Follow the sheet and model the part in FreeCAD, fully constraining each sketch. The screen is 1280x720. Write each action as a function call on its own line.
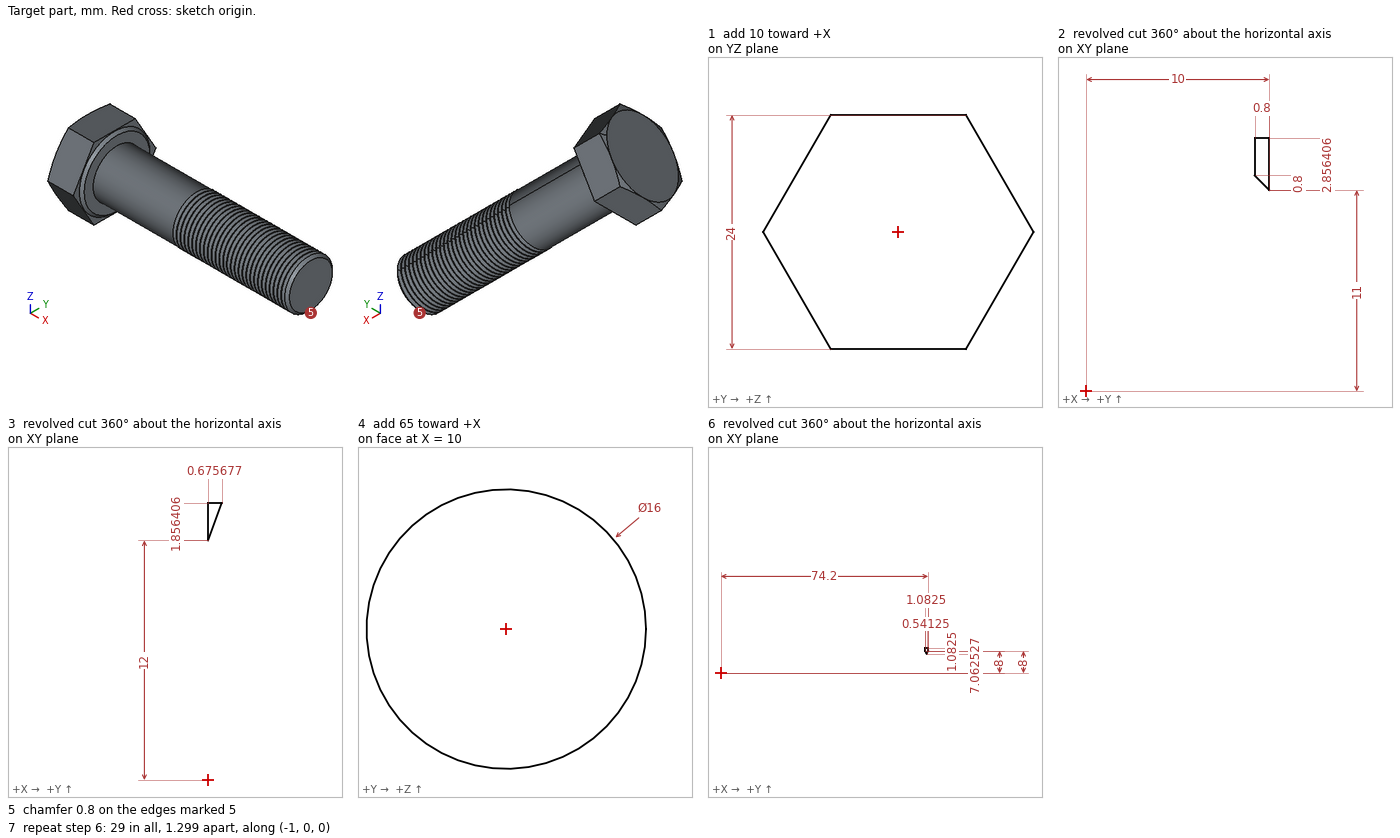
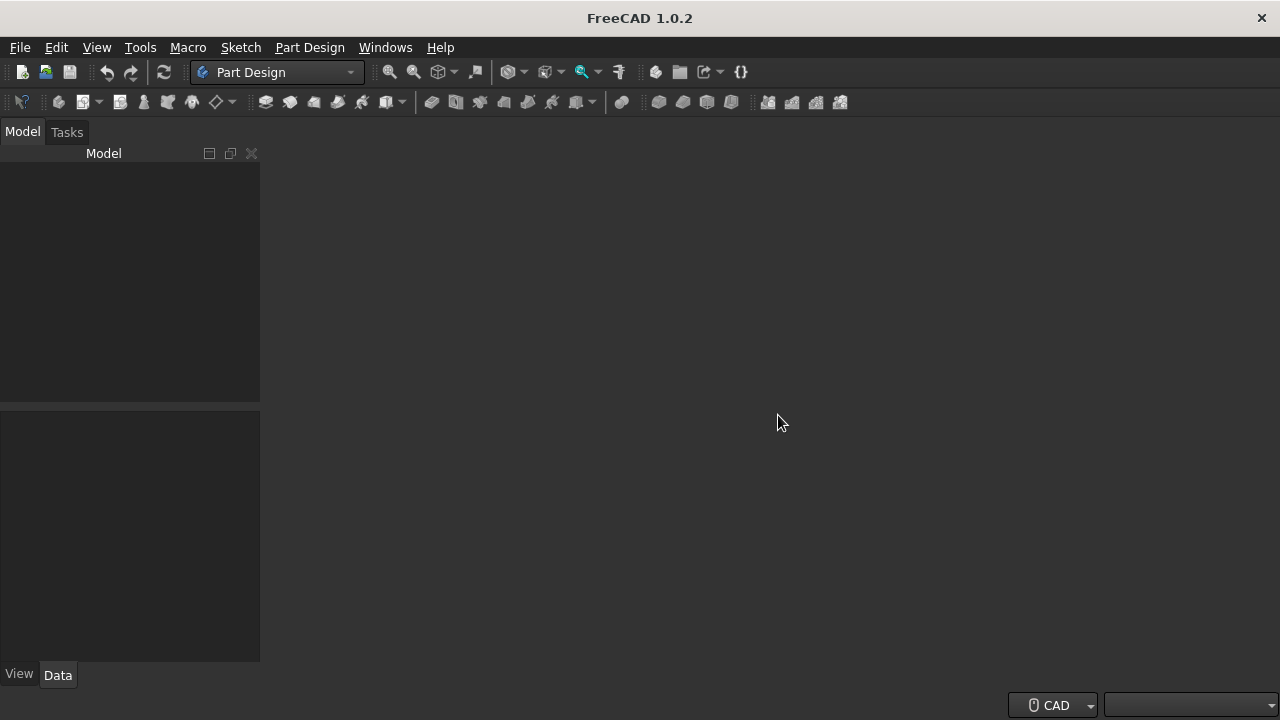
click(22, 72)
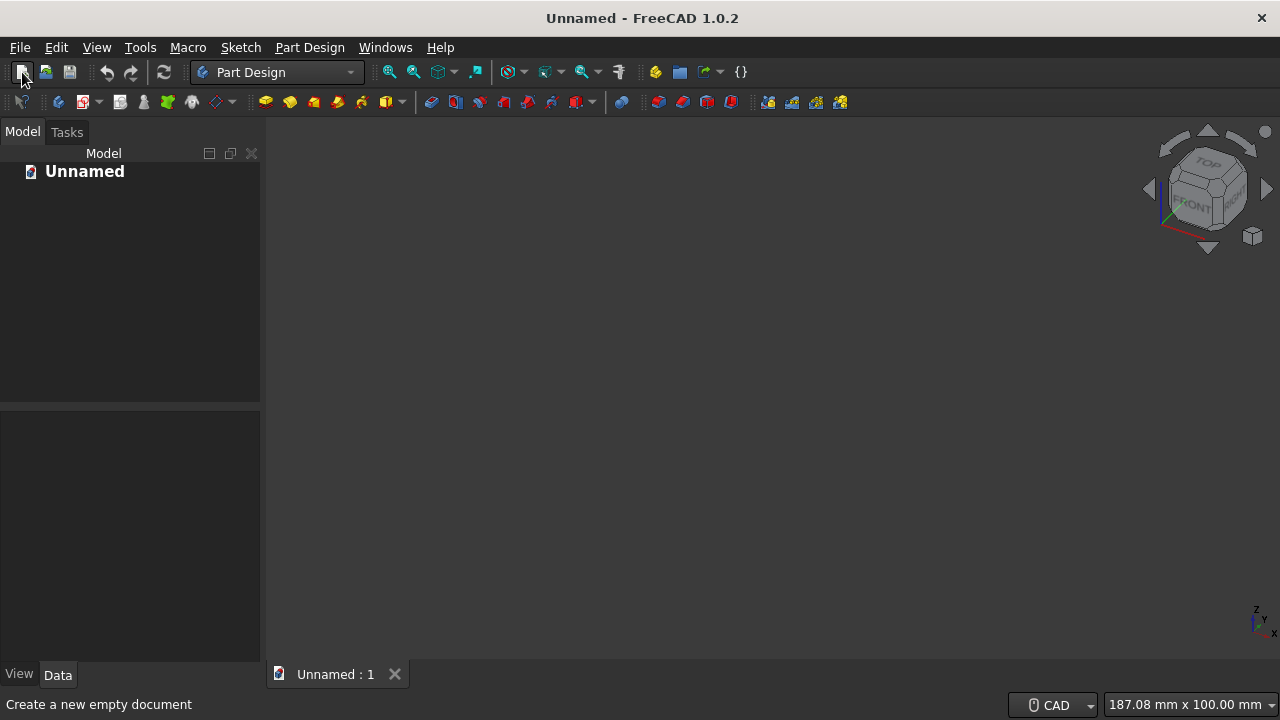
click(84, 102)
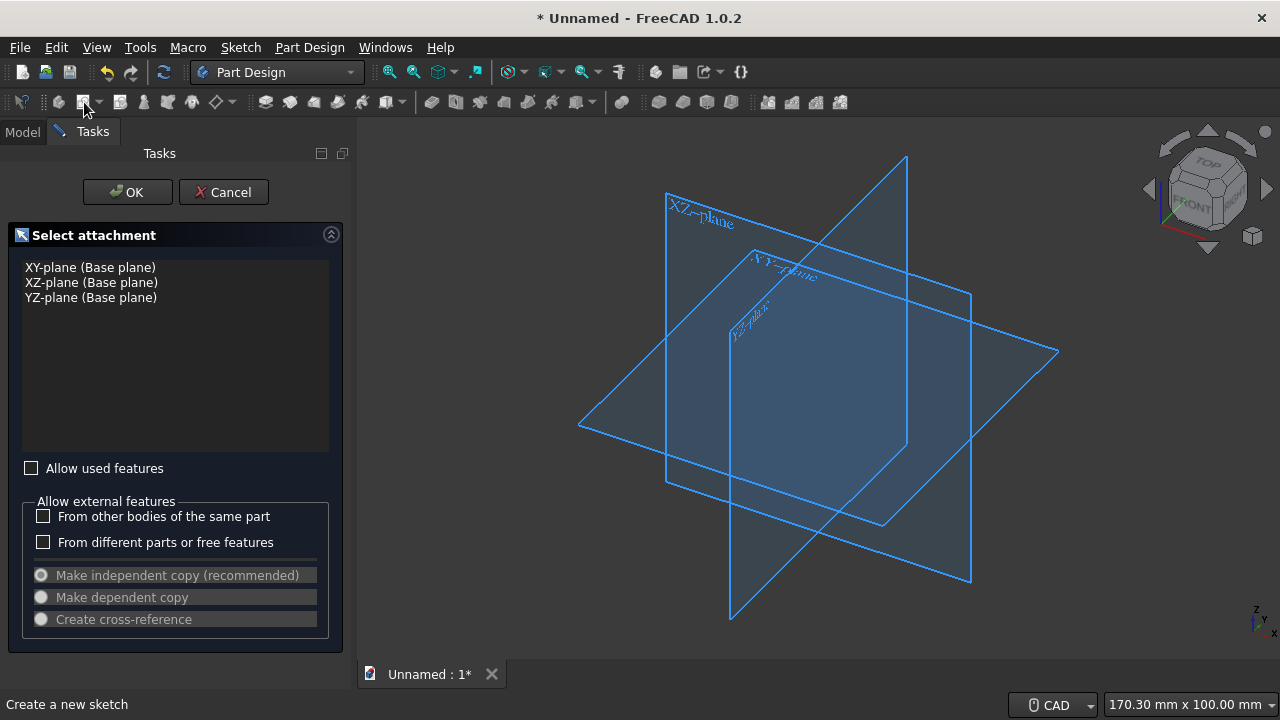
click(82, 298)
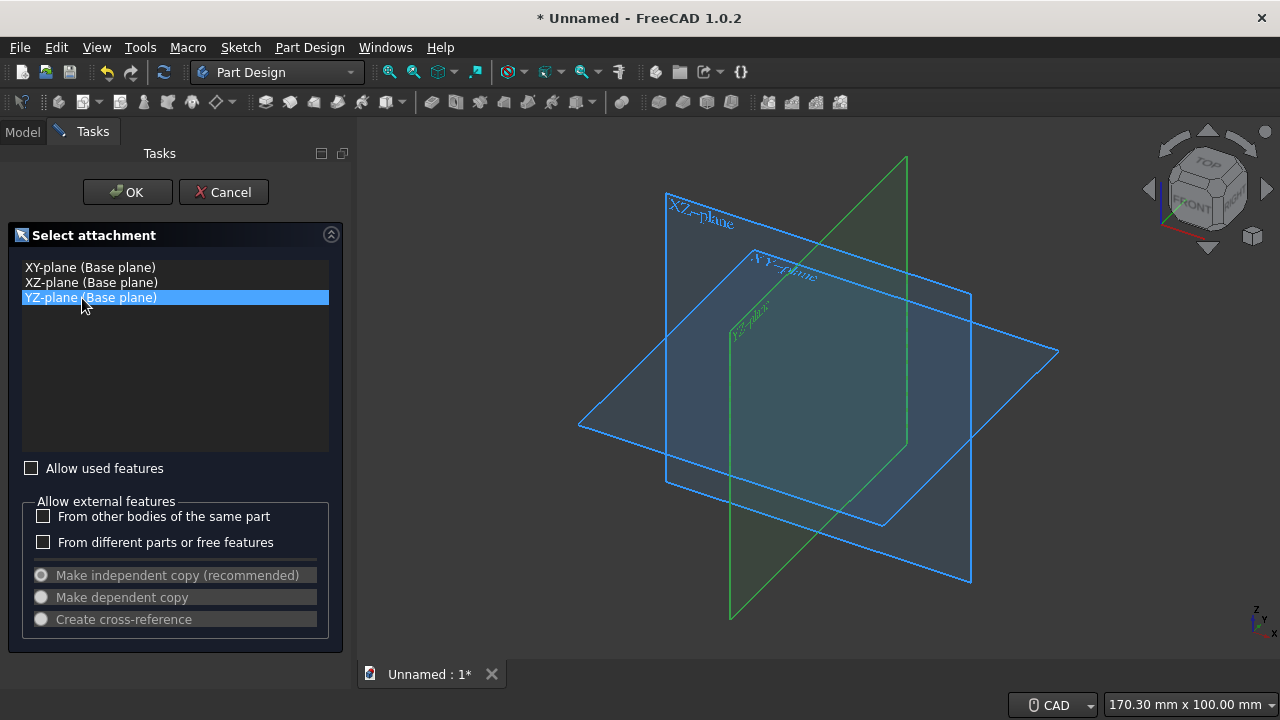
click(128, 192)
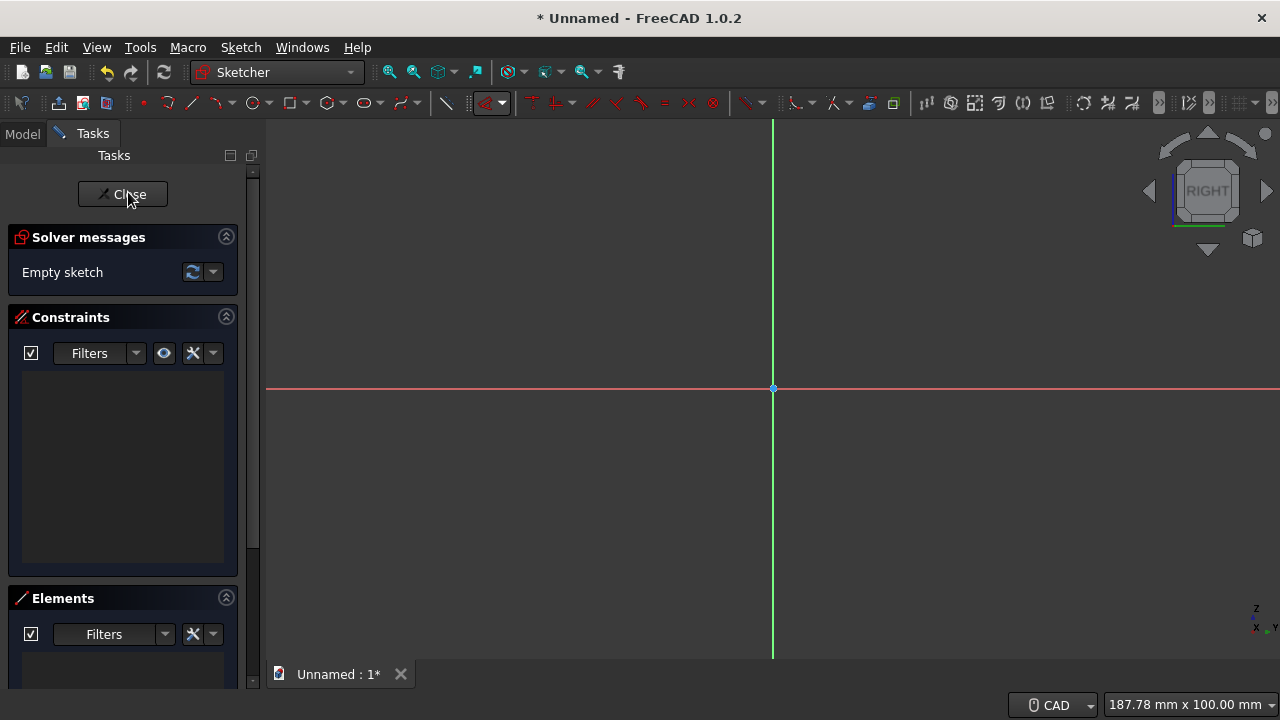
scroll(813, 389, up, 5)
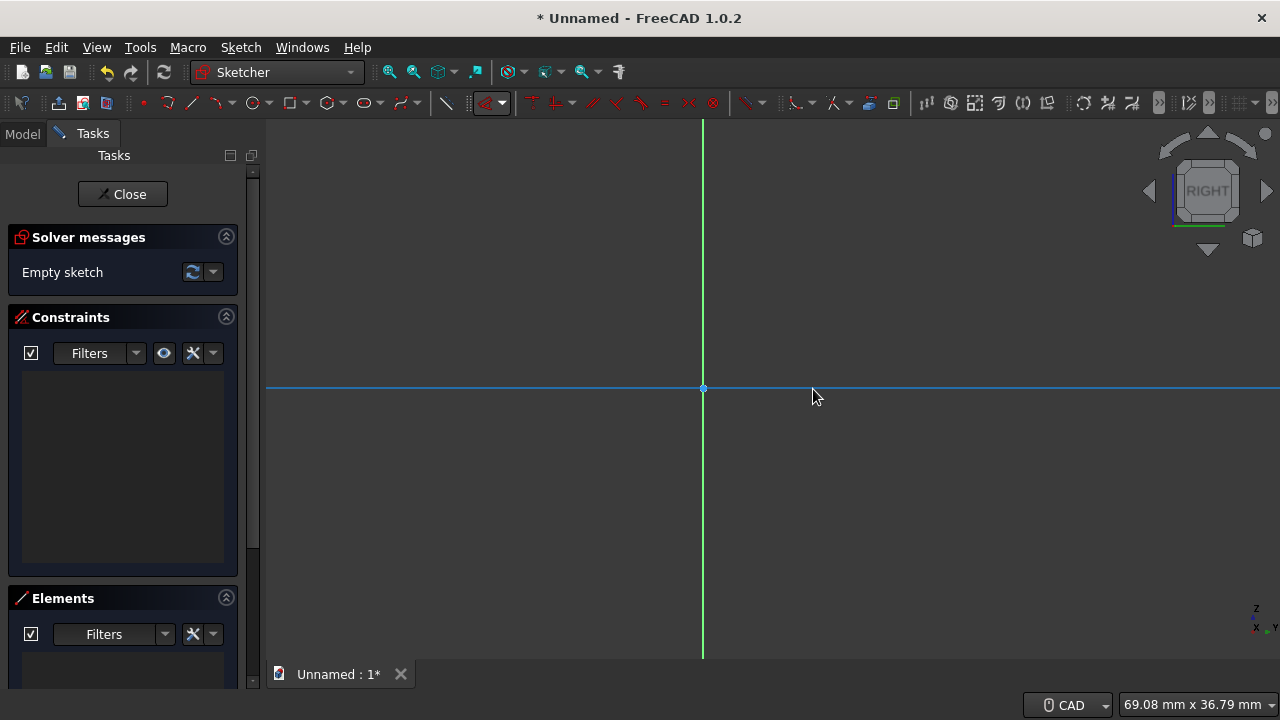
key(g)
key(p)
key(6)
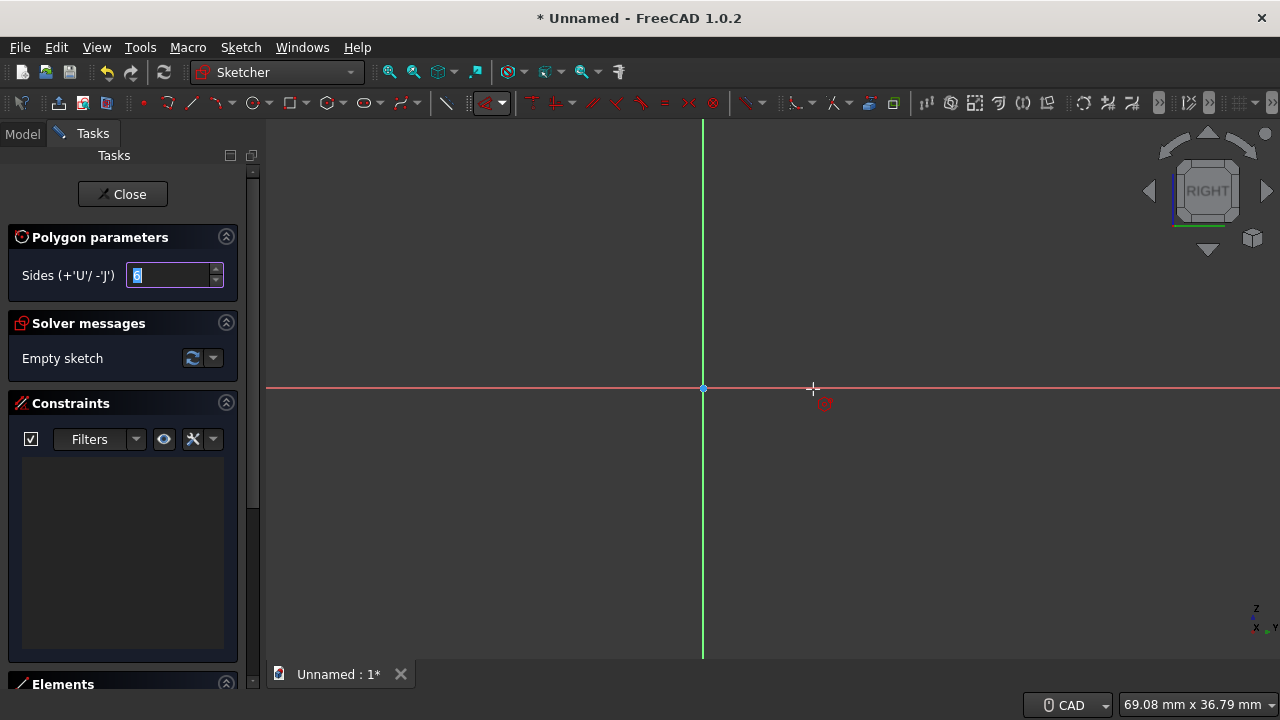
click(703, 388)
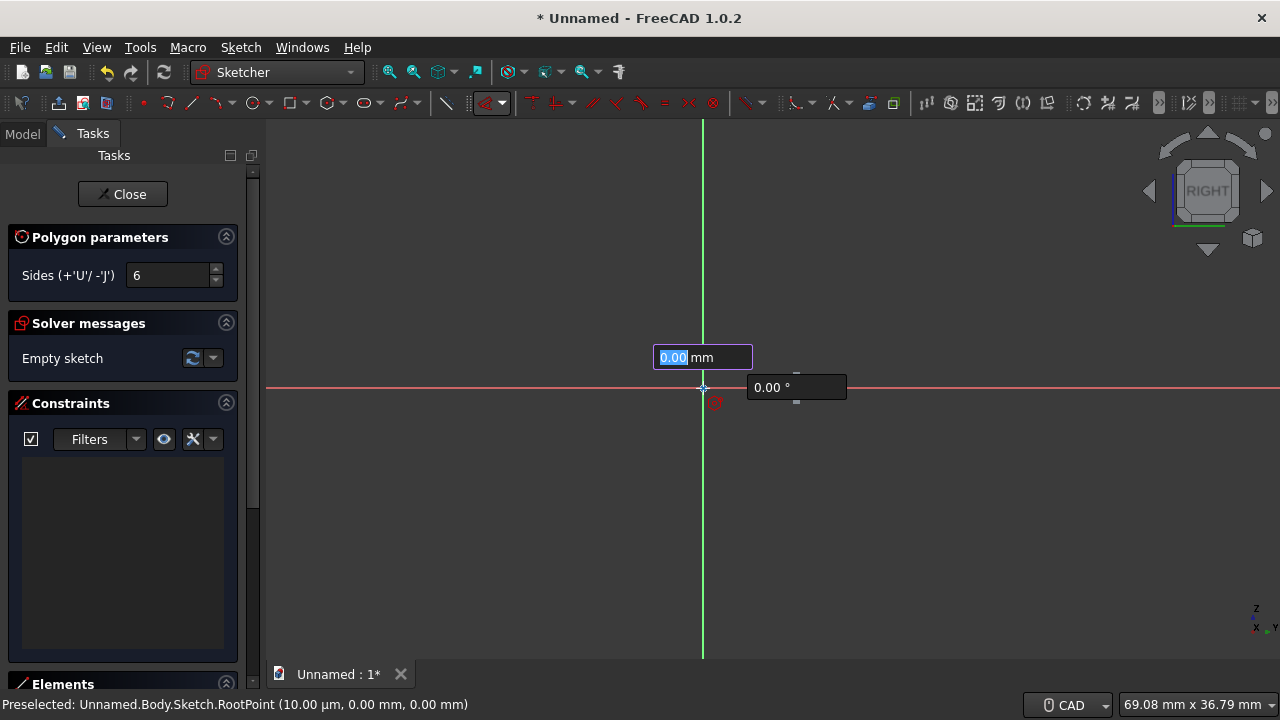
click(500, 388)
right_click(500, 388)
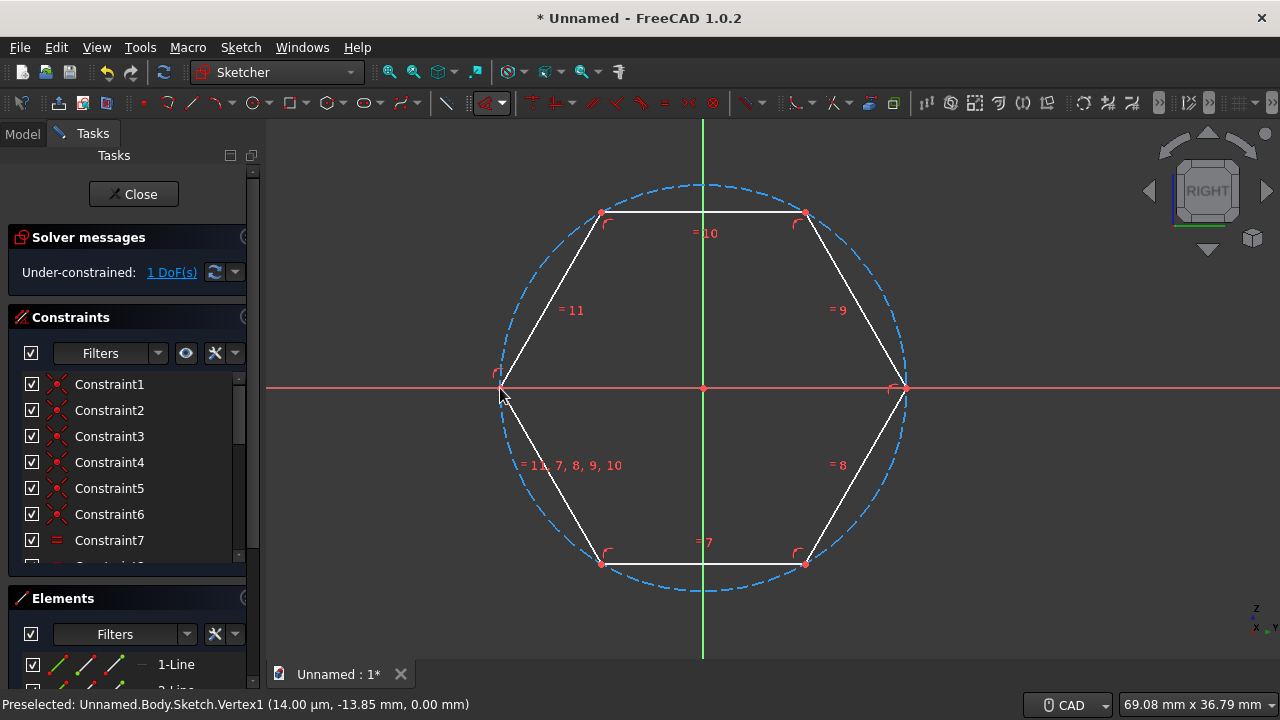
click(486, 104)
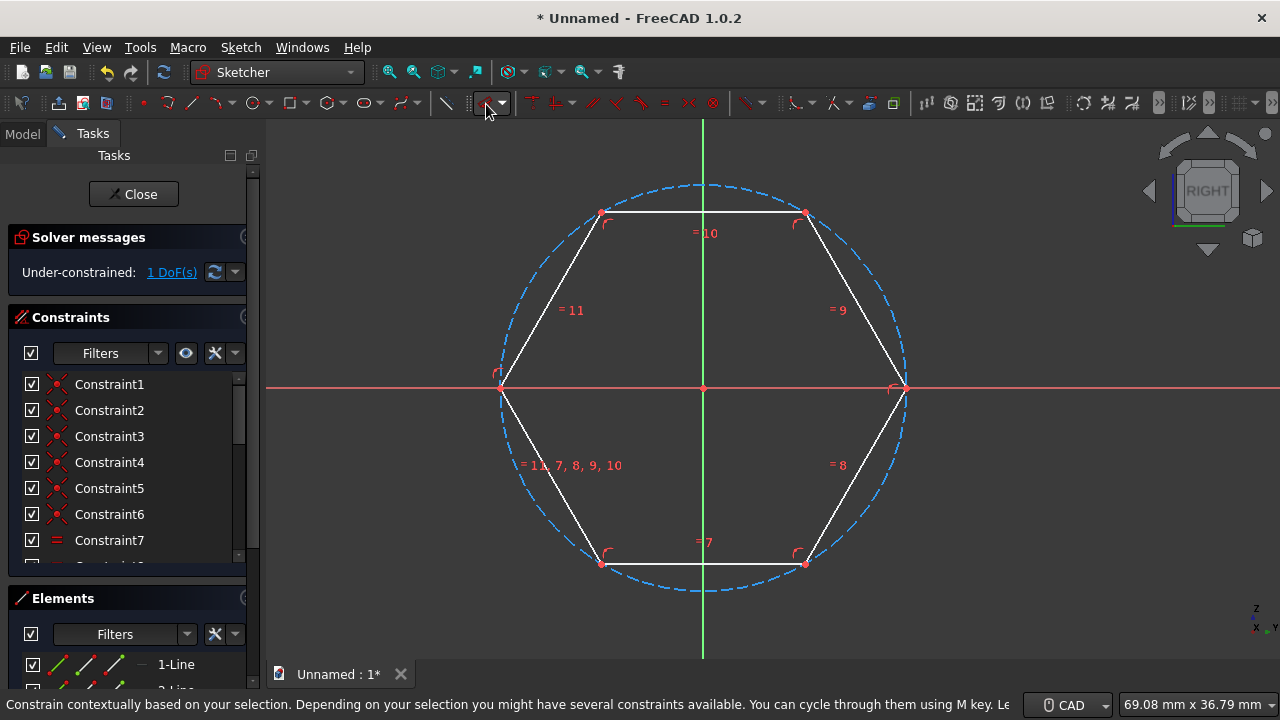
click(602, 564)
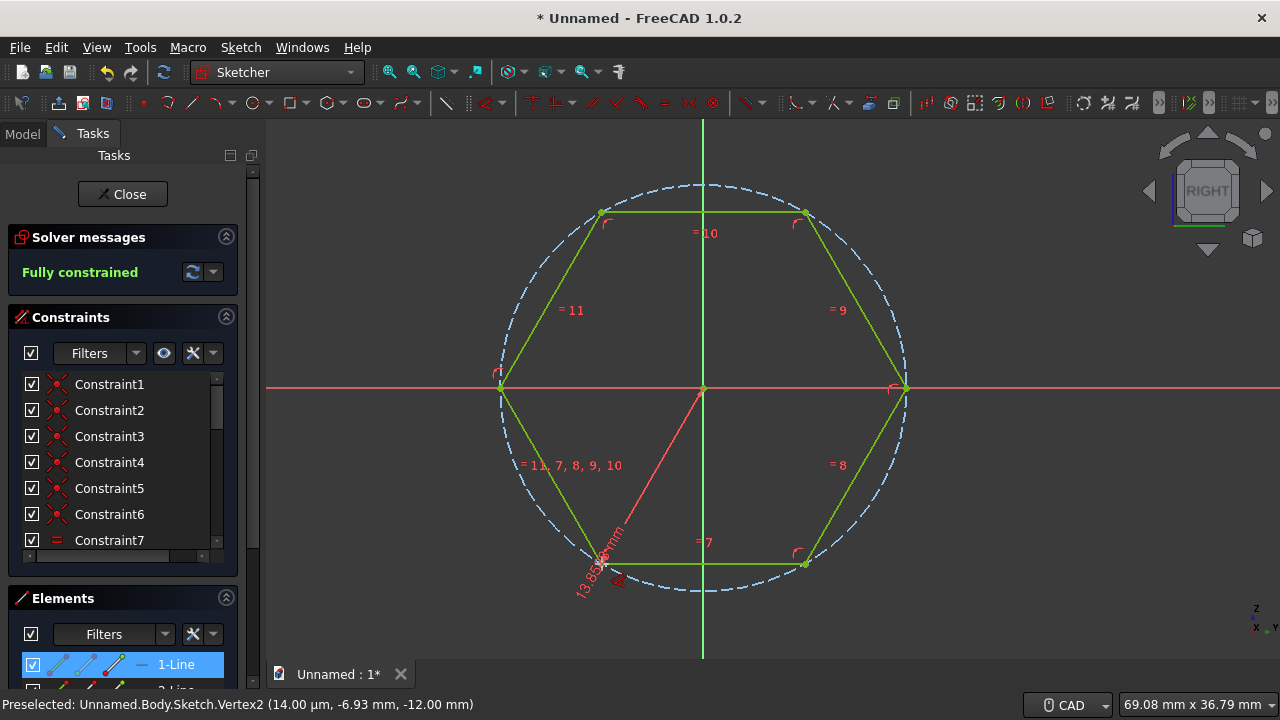
click(805, 212)
click(839, 307)